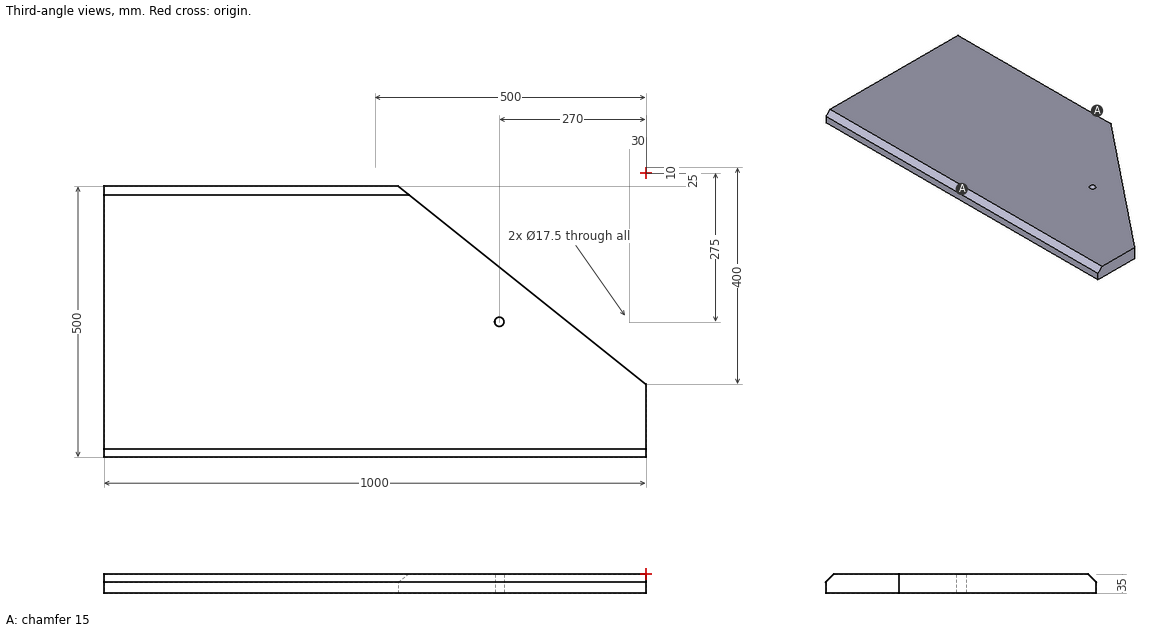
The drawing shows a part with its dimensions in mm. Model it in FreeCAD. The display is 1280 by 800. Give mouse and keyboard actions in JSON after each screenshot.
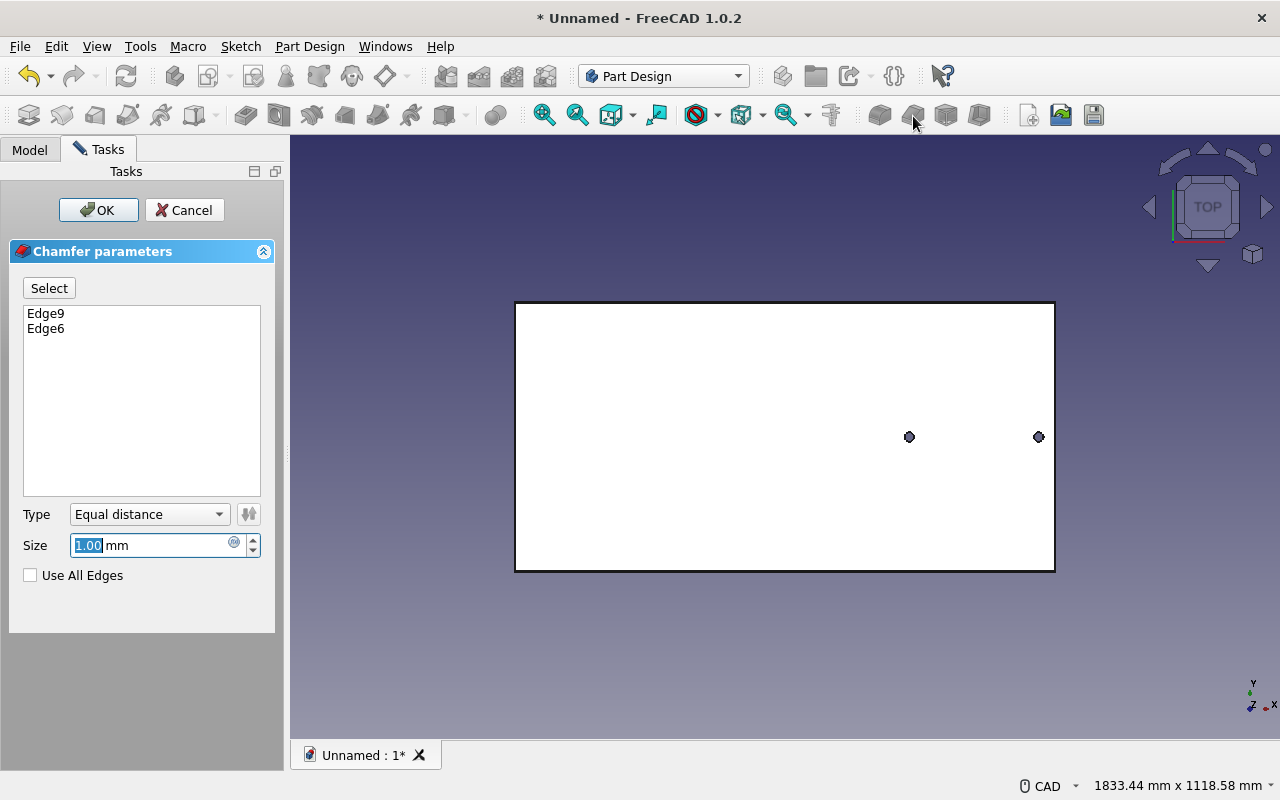
{"action": "type", "text": "15"}
{"action": "key", "text": "Tab"}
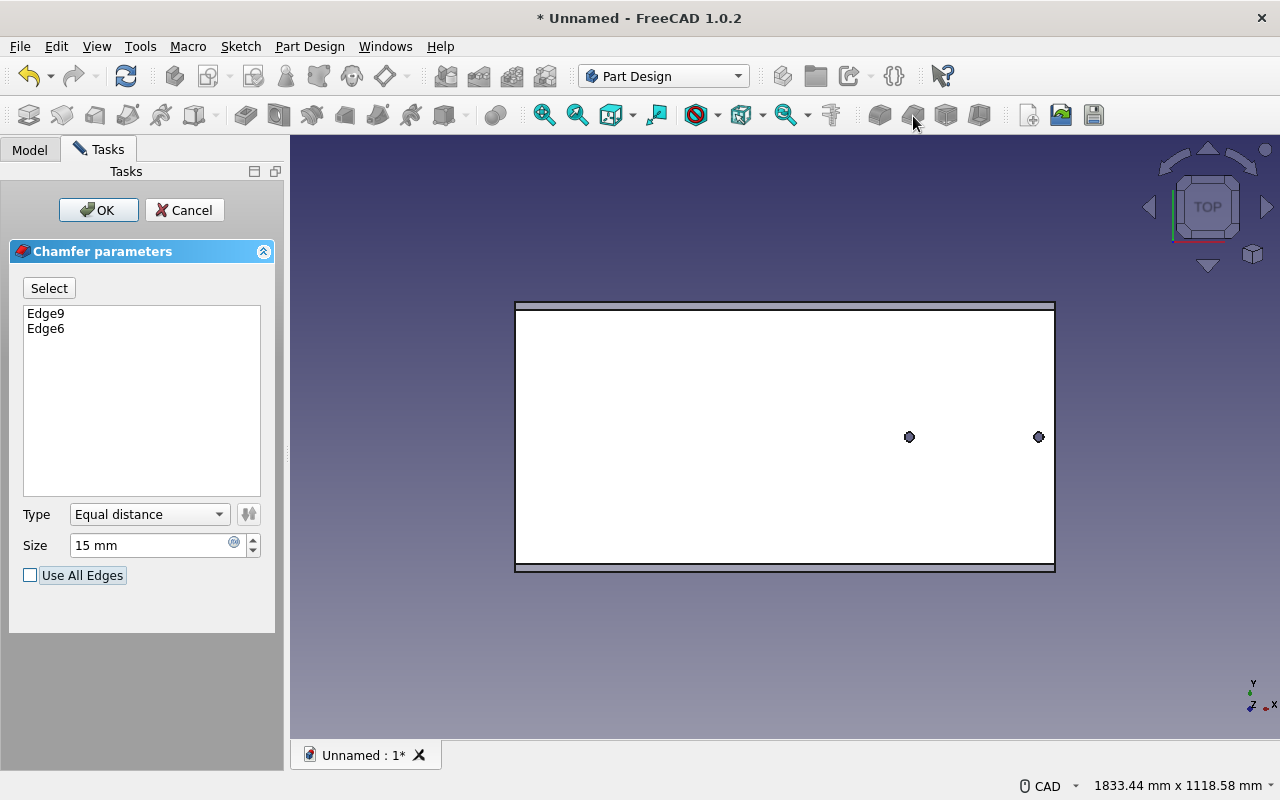
{"action": "left_click", "coordinate": [99, 210]}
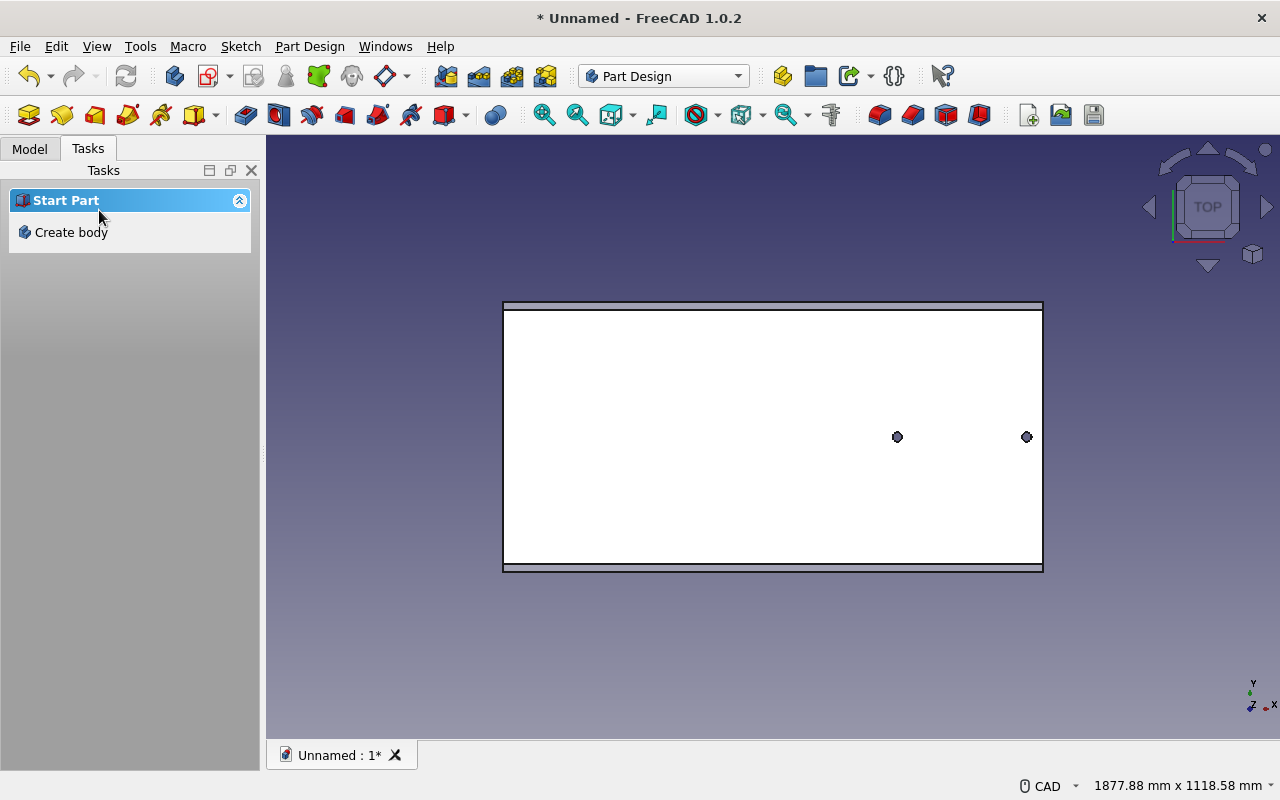
{"action": "left_click", "coordinate": [208, 76]}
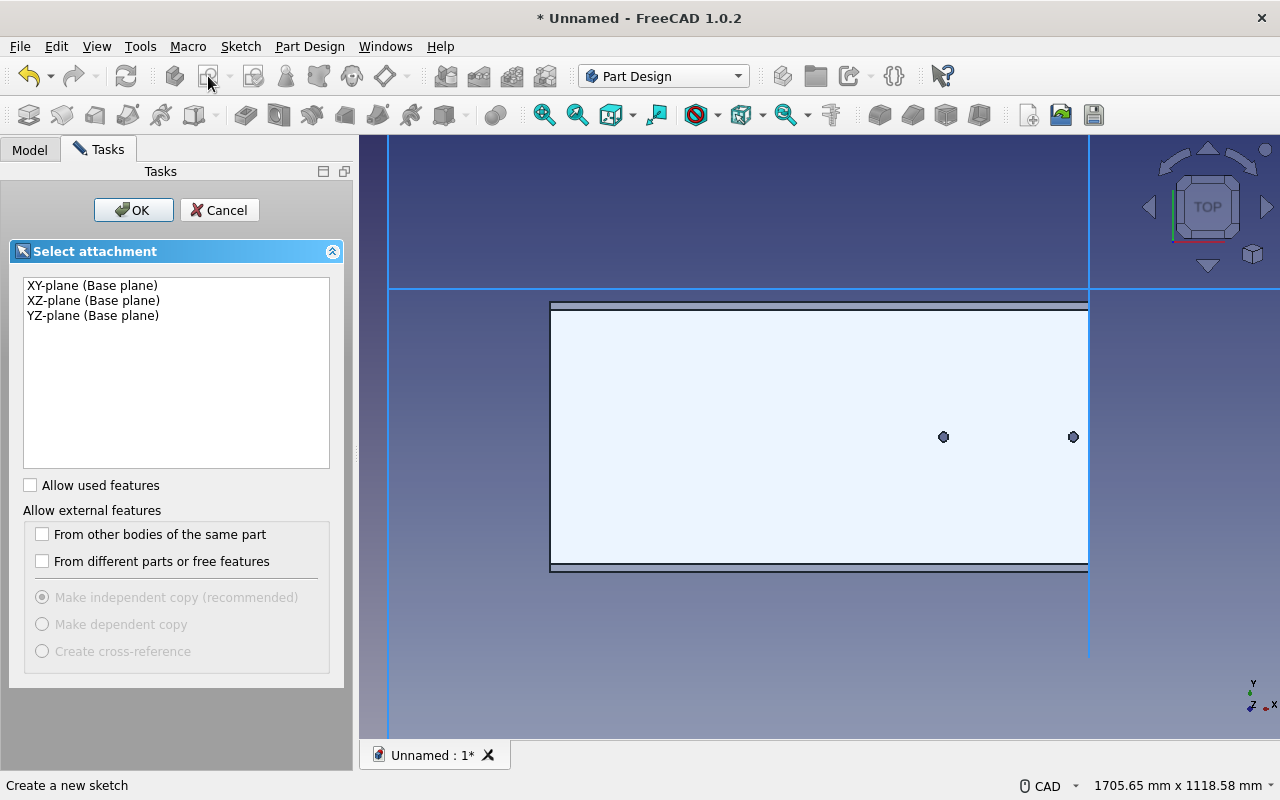
{"action": "left_click", "coordinate": [84, 286]}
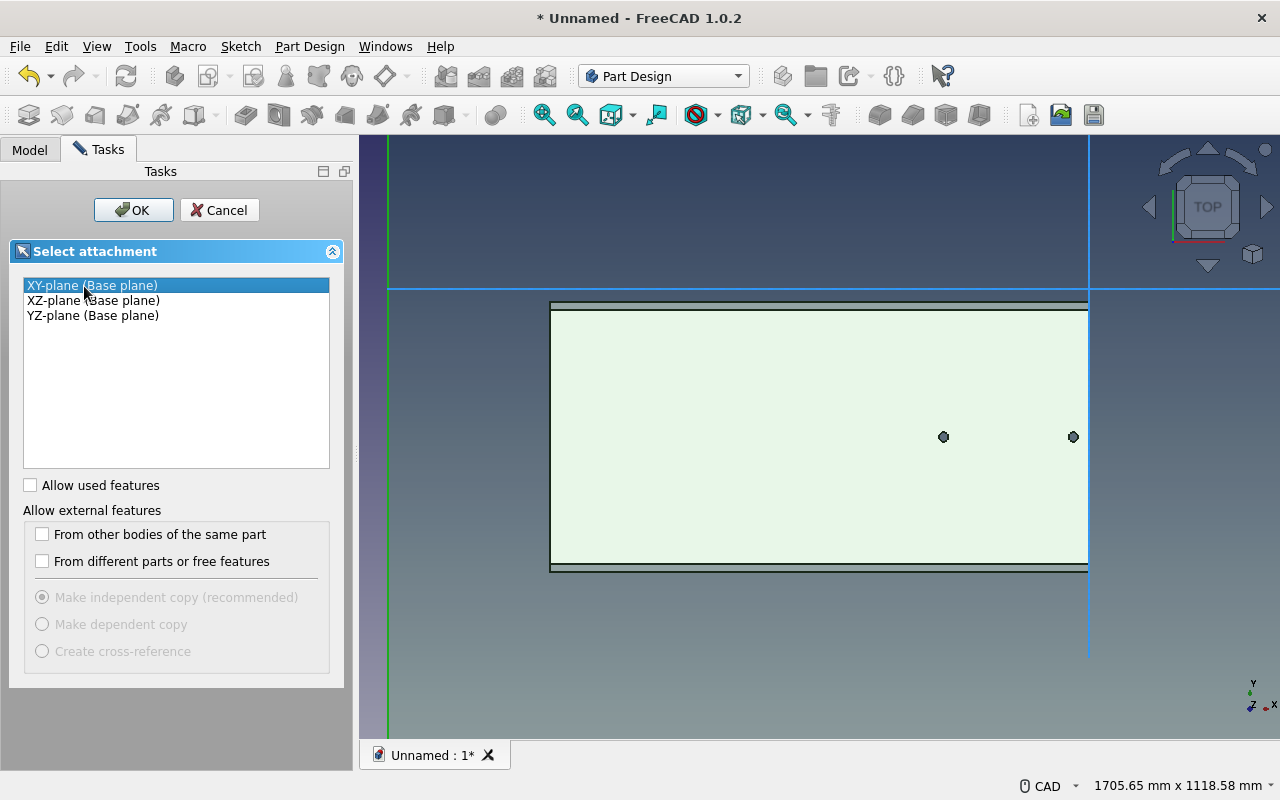
{"action": "left_click", "coordinate": [134, 210]}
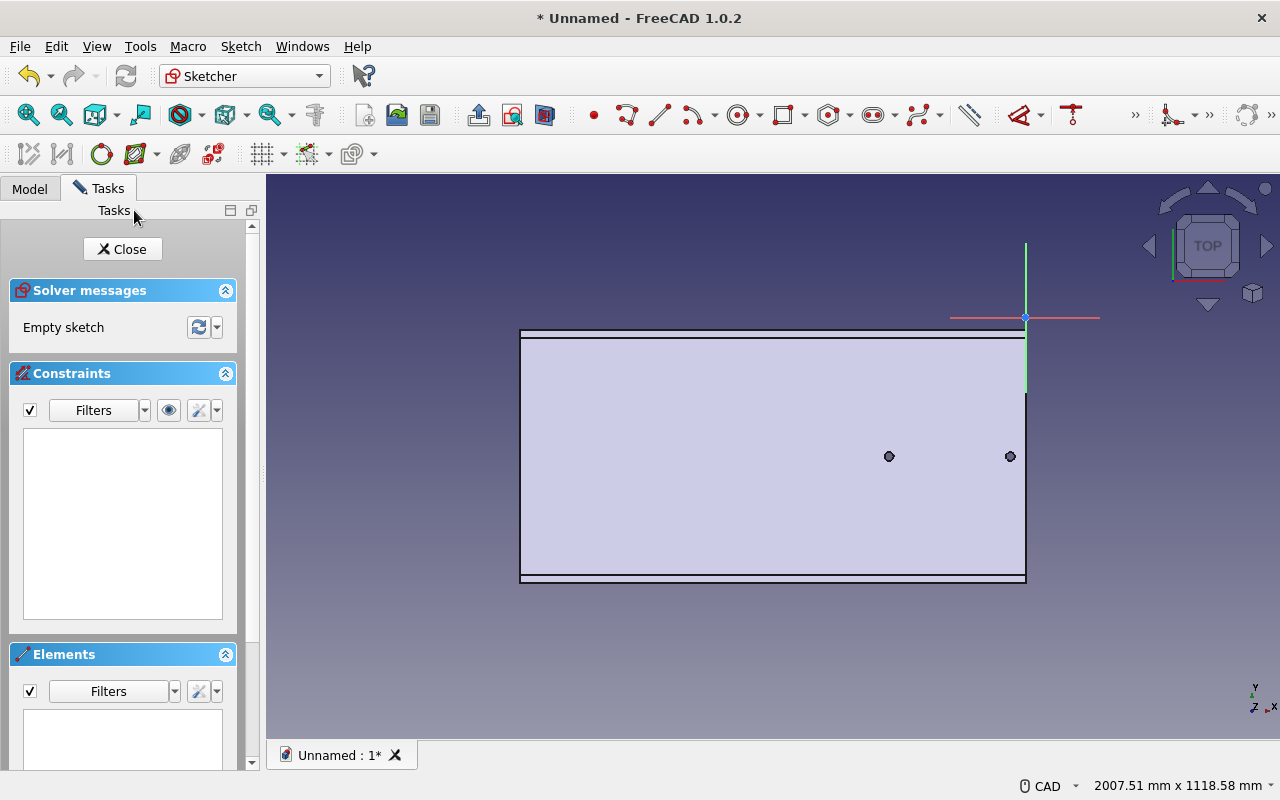
{"action": "scroll", "coordinate": [1115, 361], "scroll_direction": "up", "scroll_amount": 3}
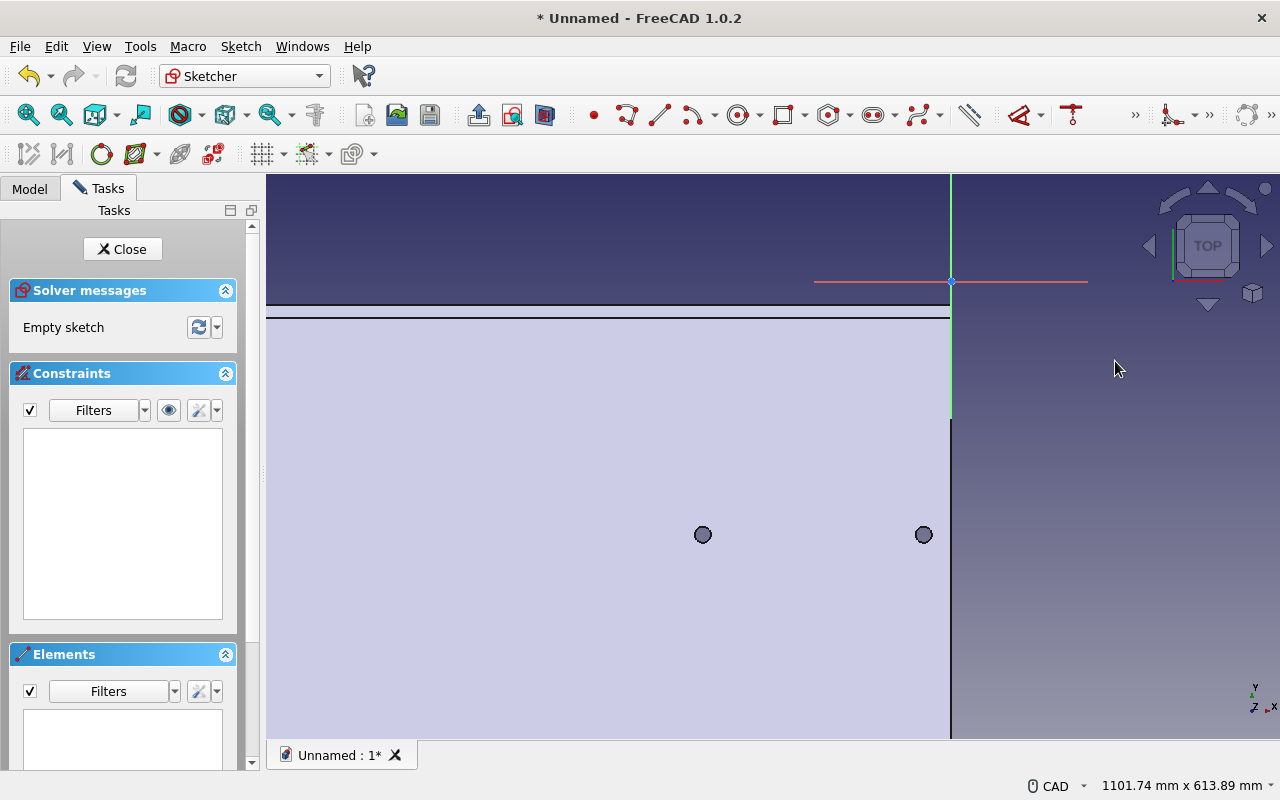
{"action": "key", "text": "g m"}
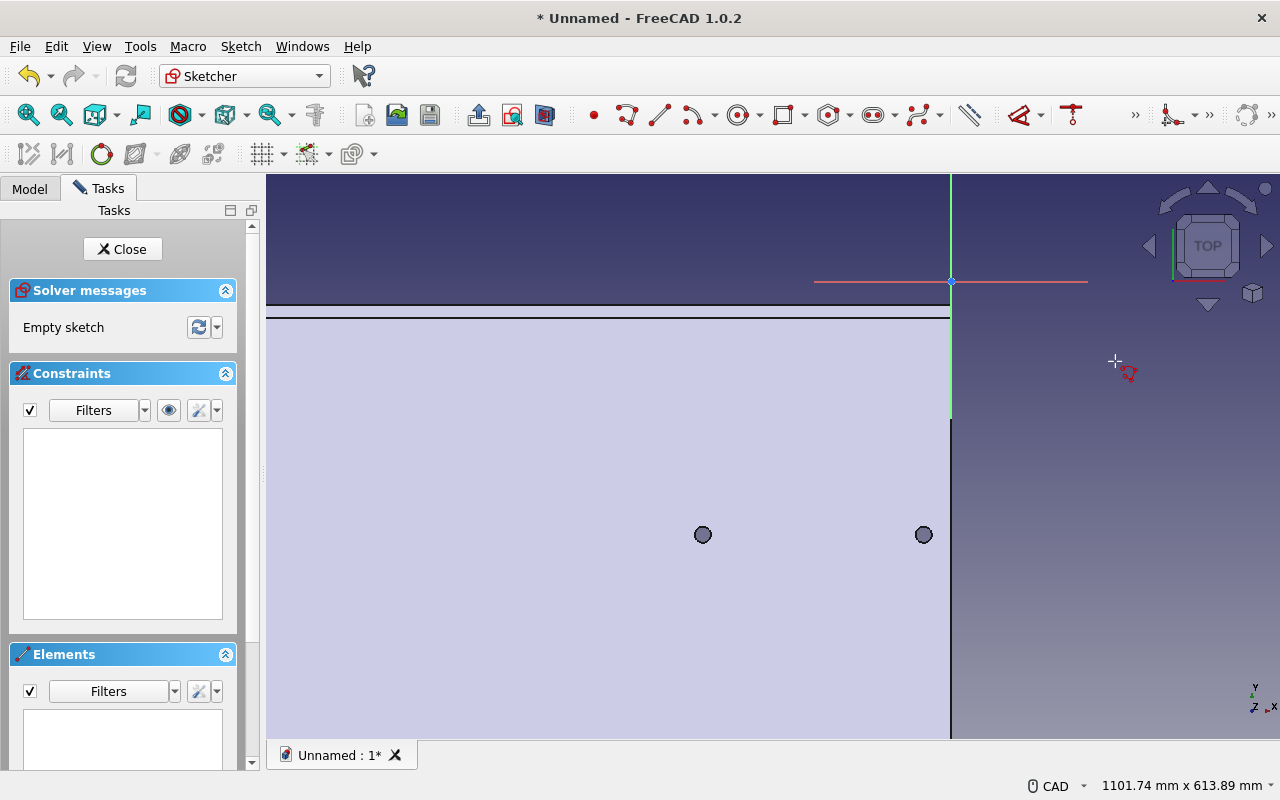
{"action": "scroll", "coordinate": [951, 272], "scroll_direction": "up", "scroll_amount": 3}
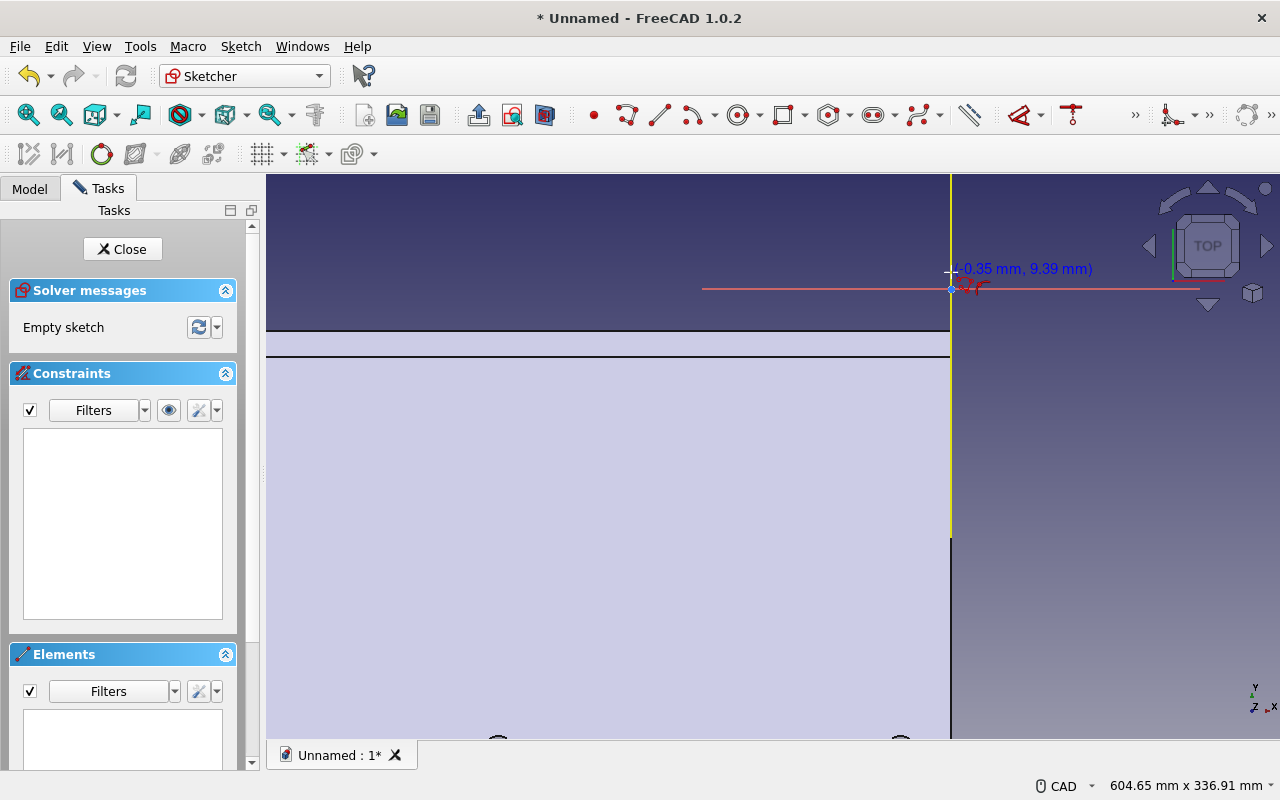
{"action": "left_click", "coordinate": [951, 273]}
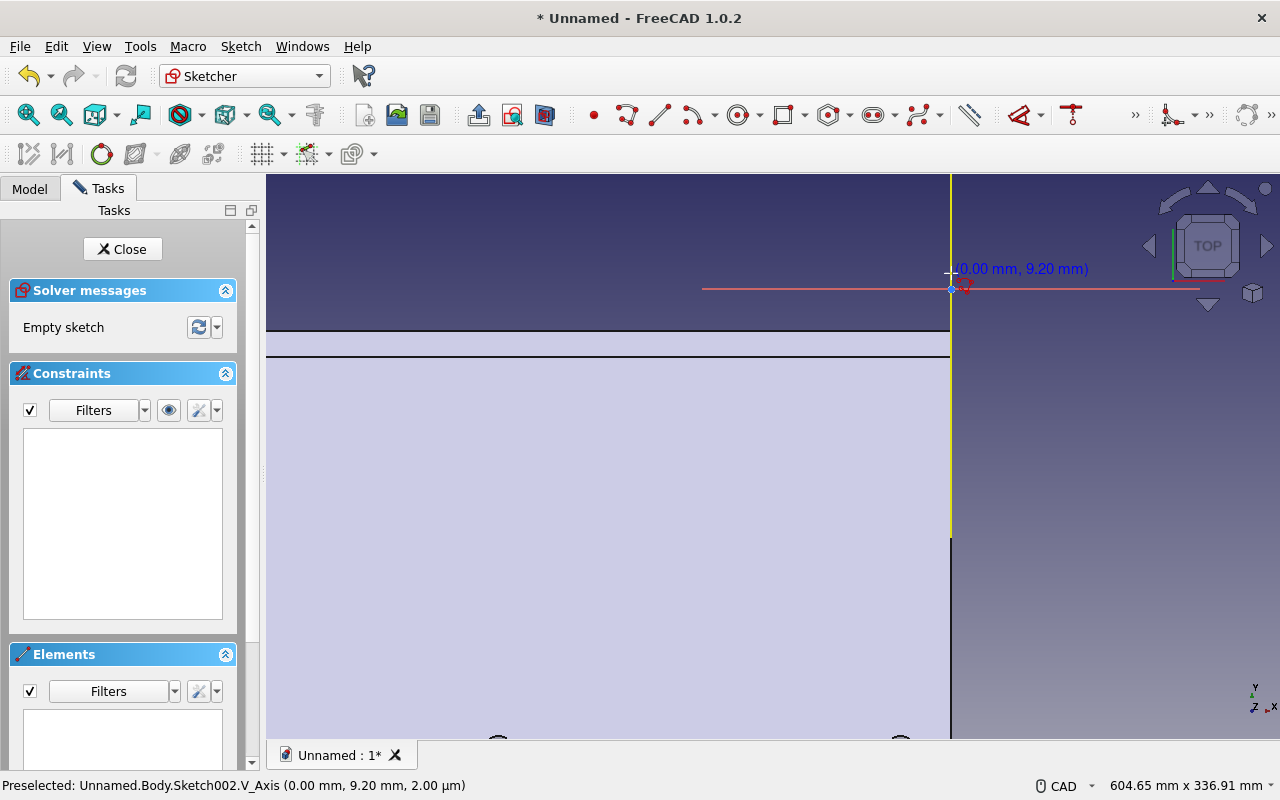
{"action": "scroll", "coordinate": [915, 272], "scroll_direction": "down", "scroll_amount": 3}